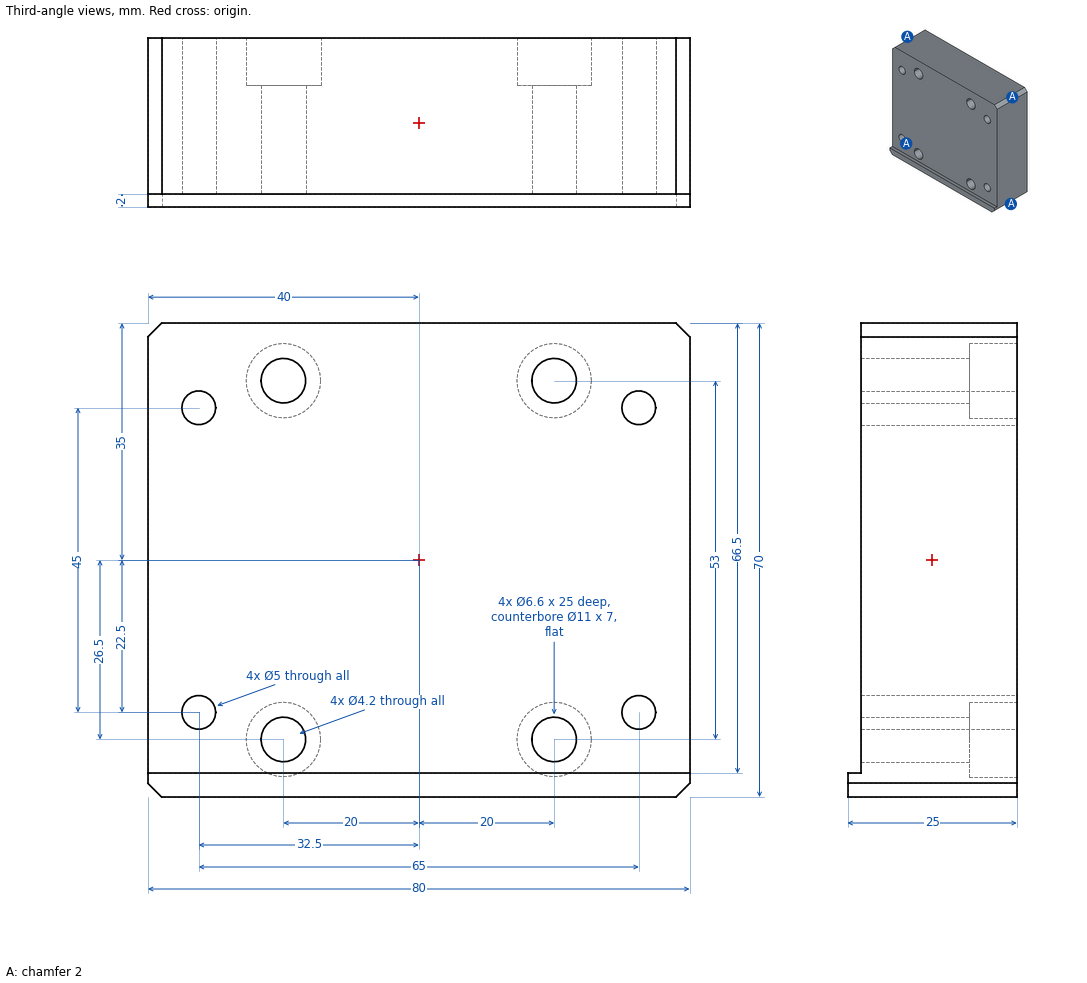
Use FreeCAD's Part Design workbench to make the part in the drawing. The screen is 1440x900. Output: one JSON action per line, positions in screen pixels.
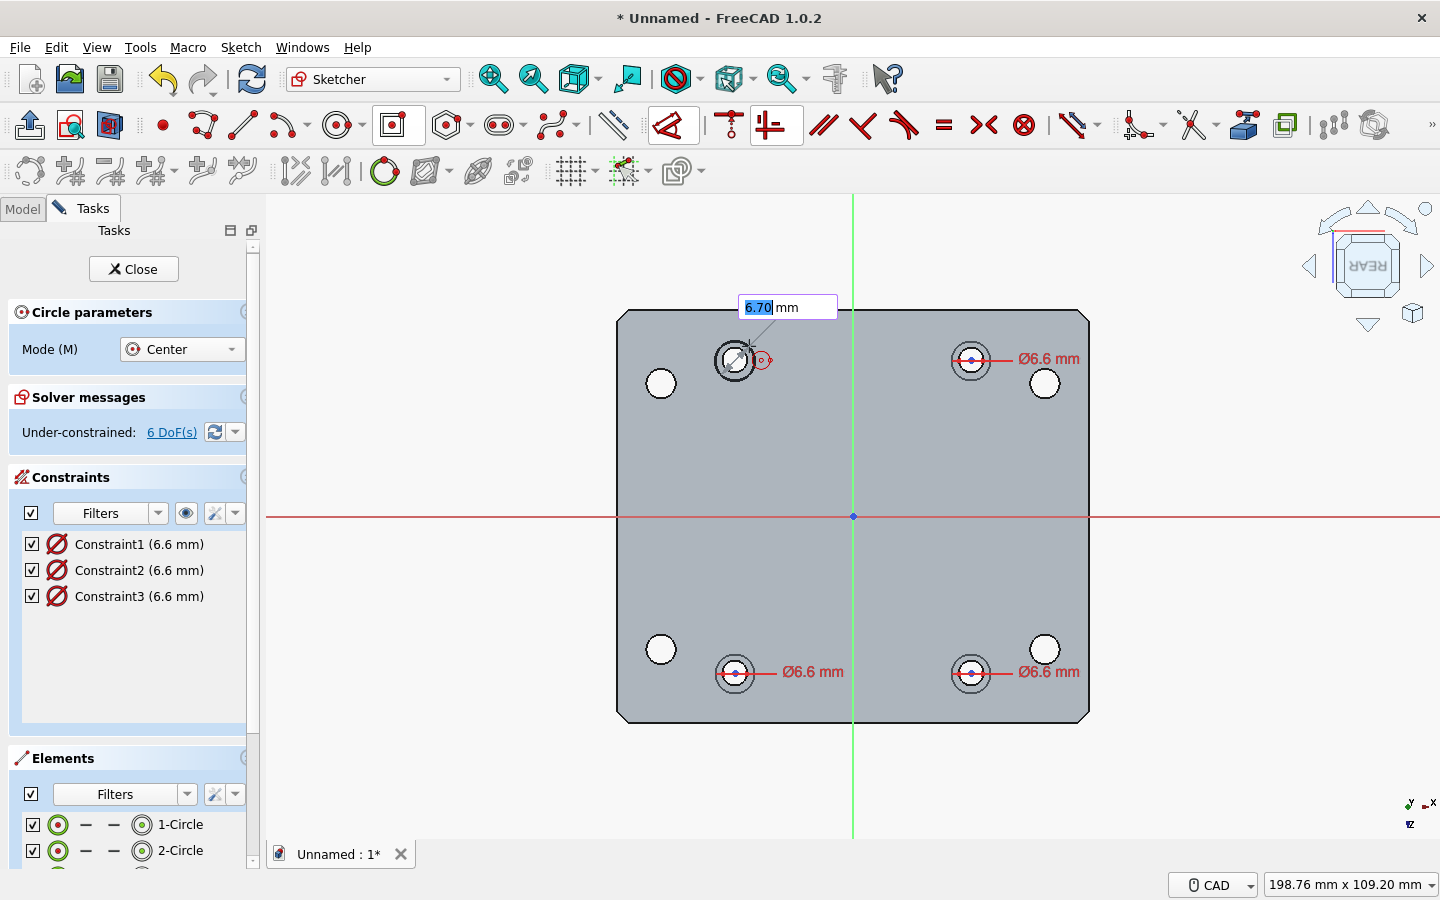
{"action": "type", "text": "6.6"}
{"action": "key", "text": "Return"}
{"action": "key", "text": "Escape"}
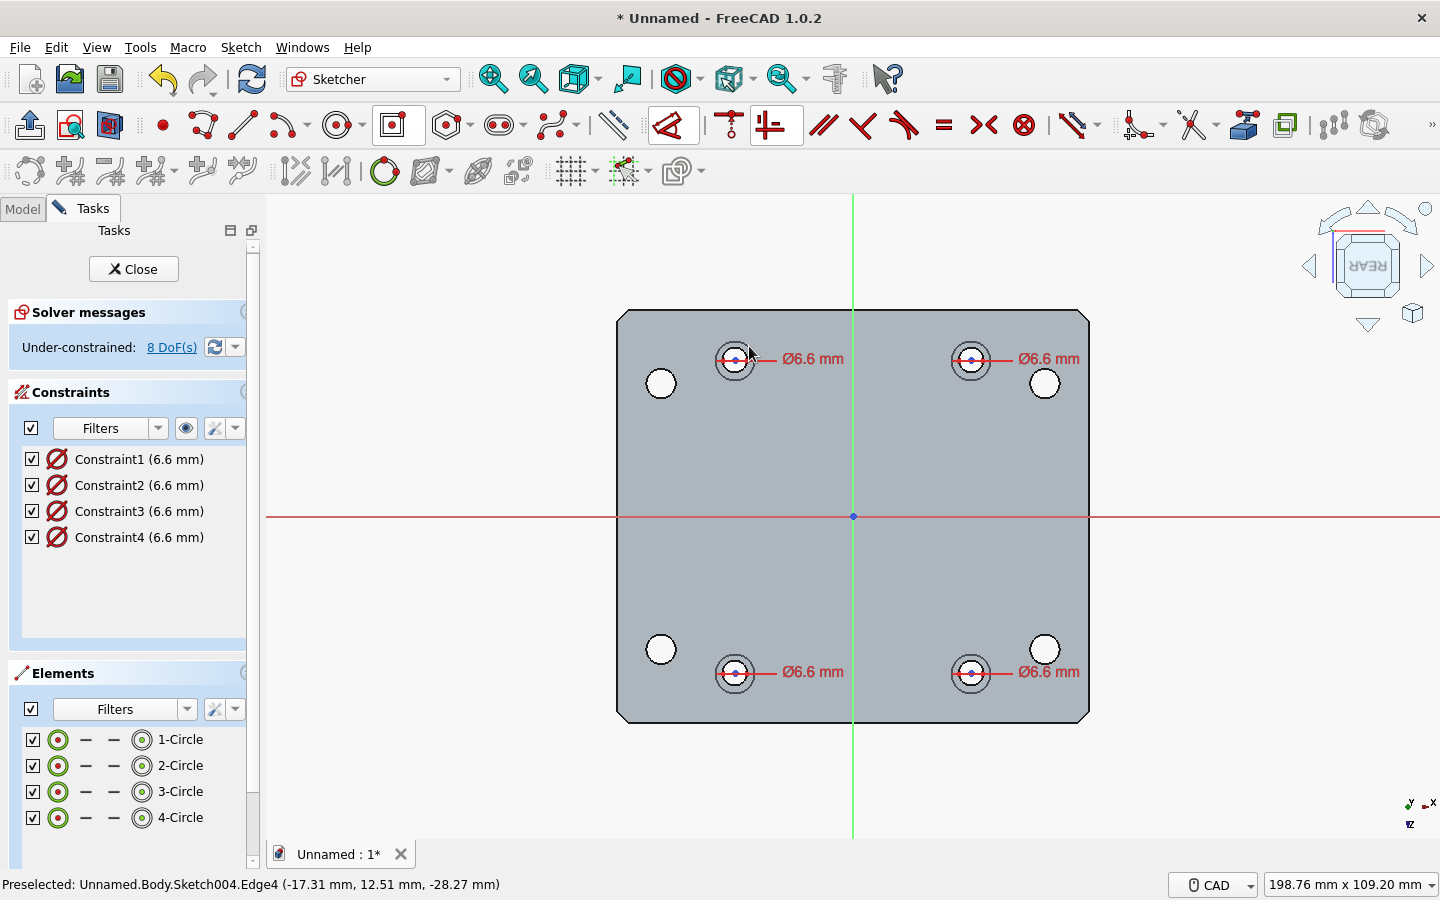
{"action": "left_click", "coordinate": [971, 361]}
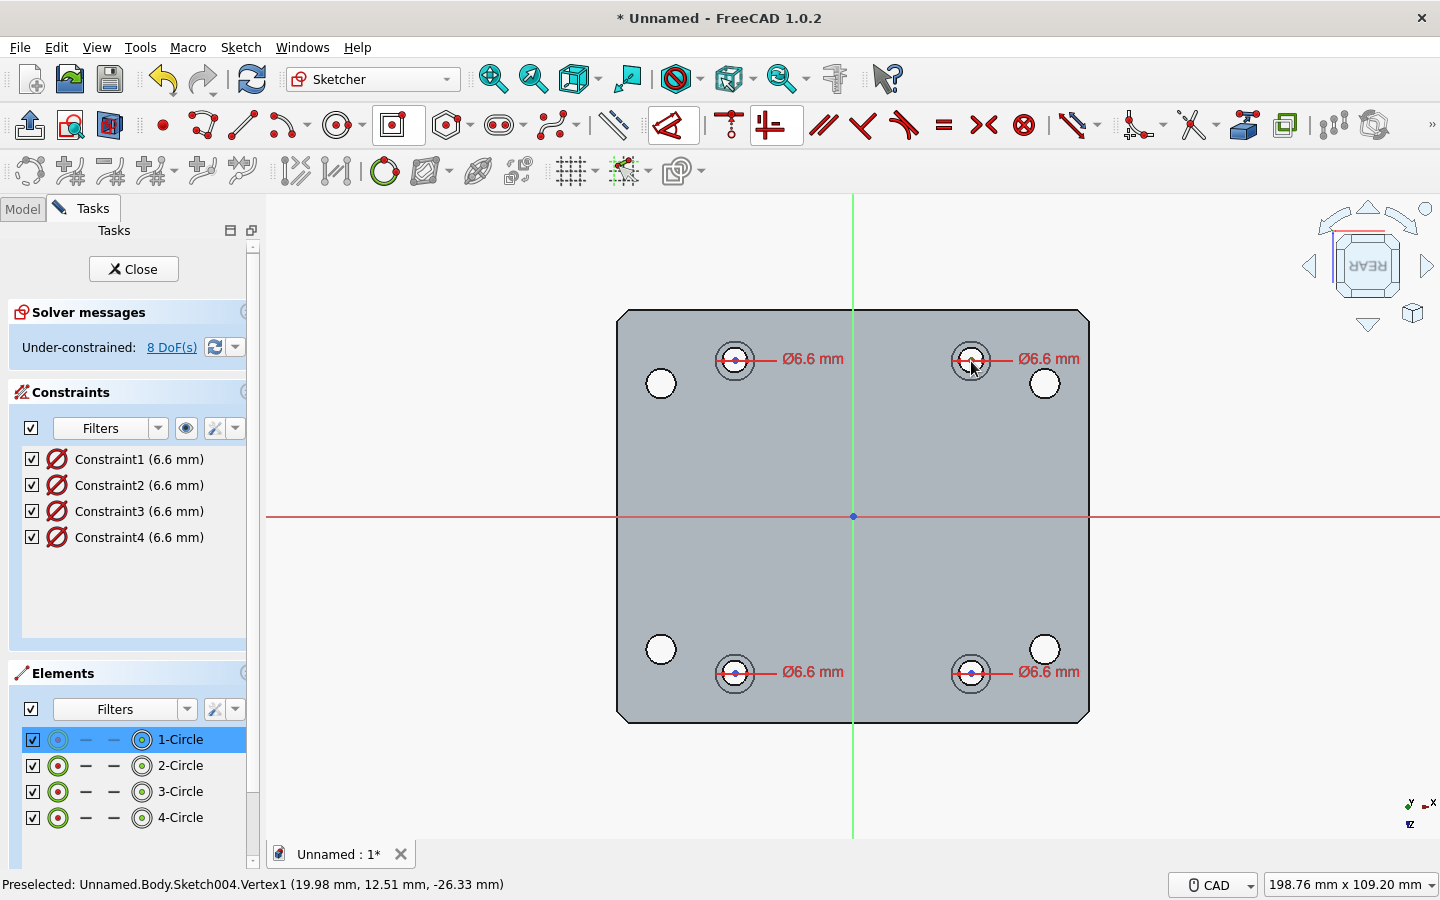
{"action": "left_click", "coordinate": [971, 674]}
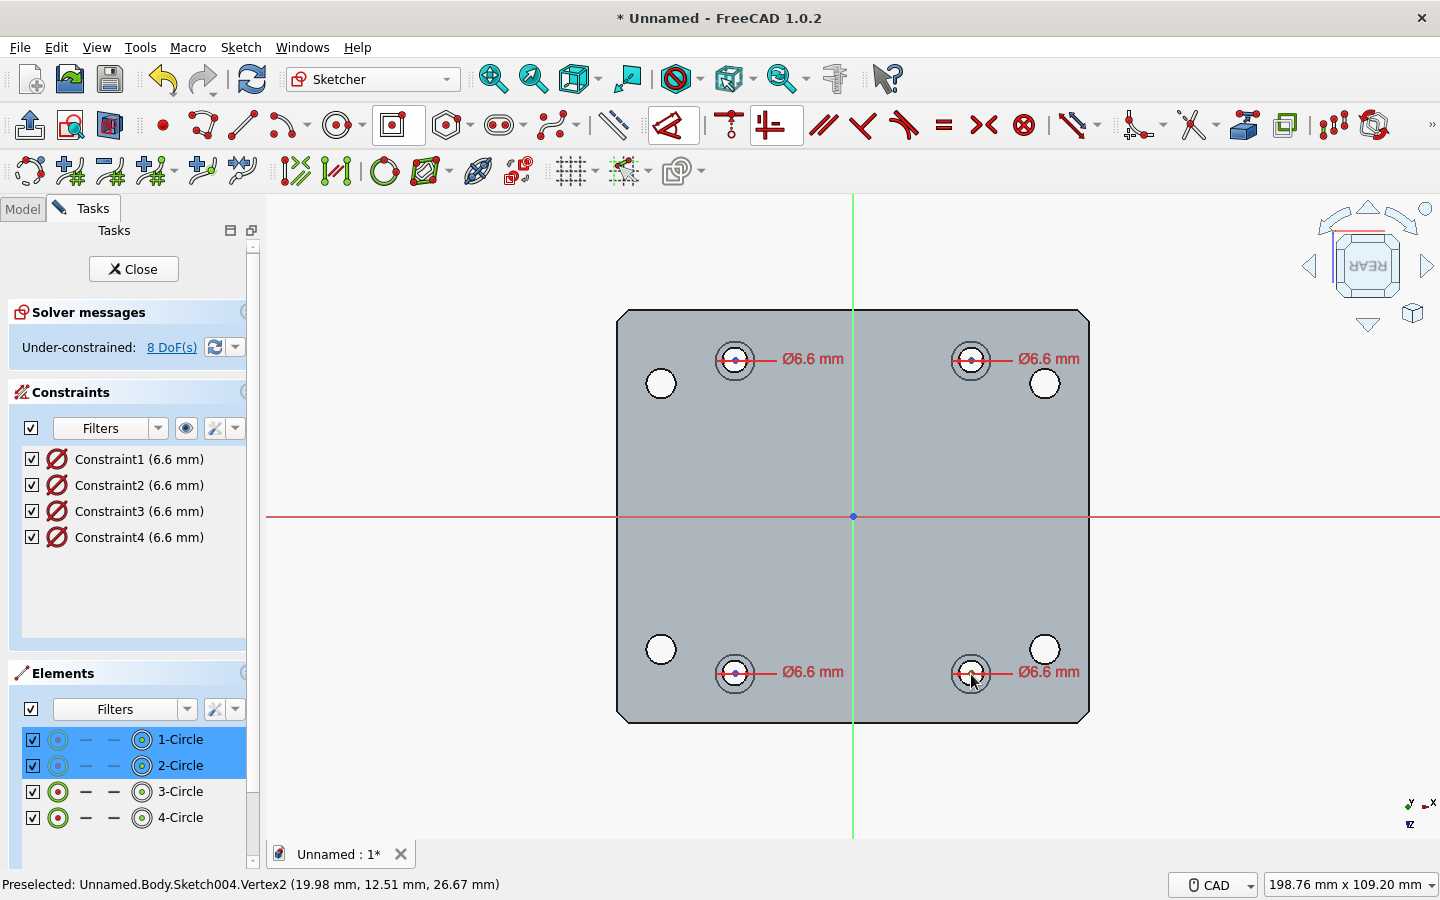
{"action": "key", "text": "v"}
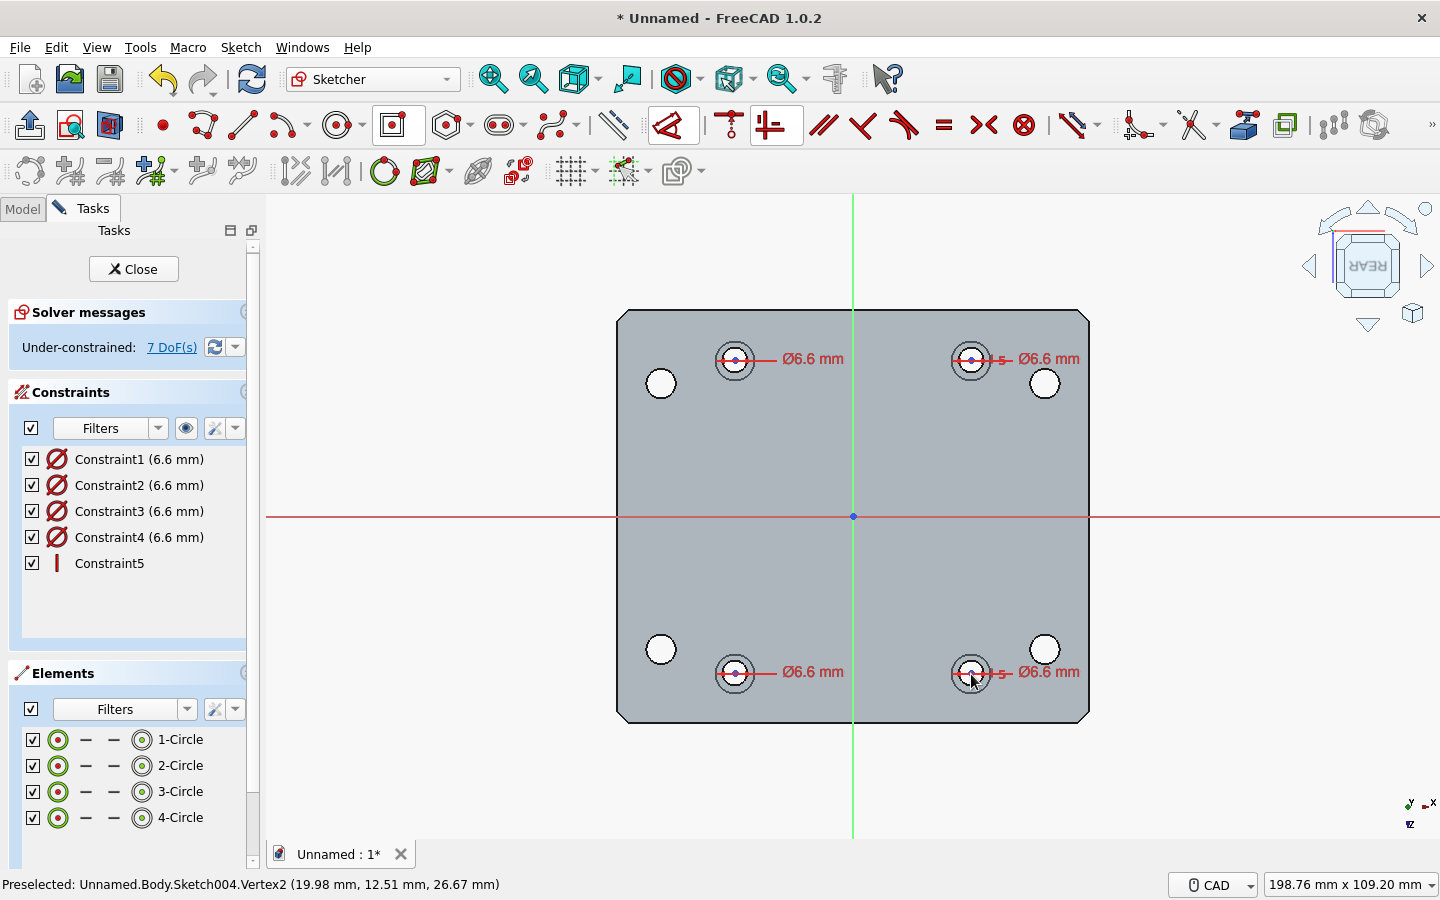
{"action": "left_click", "coordinate": [971, 674]}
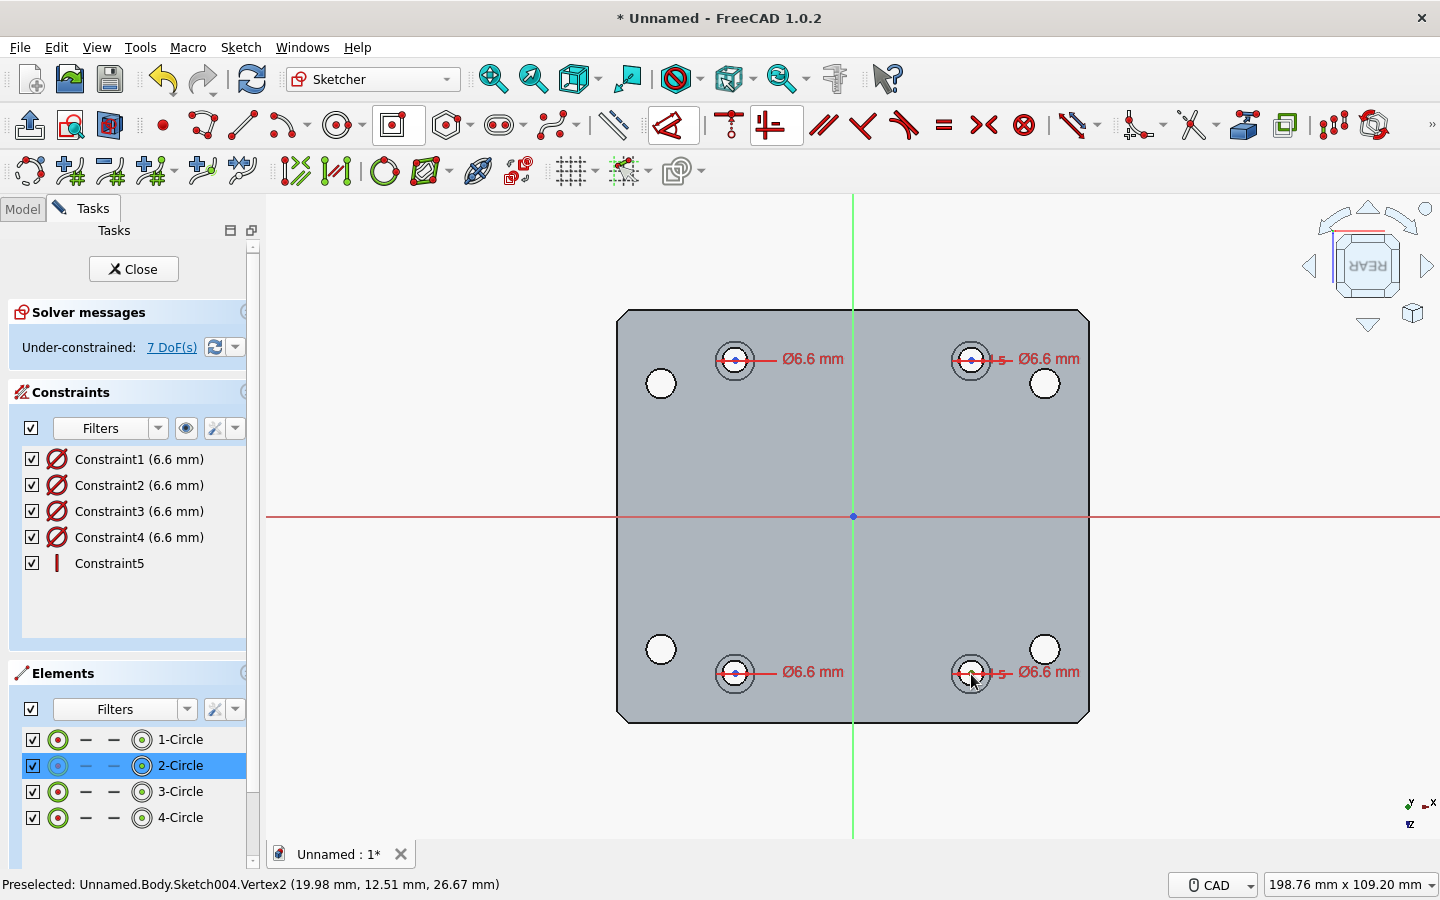
{"action": "left_click", "coordinate": [735, 674]}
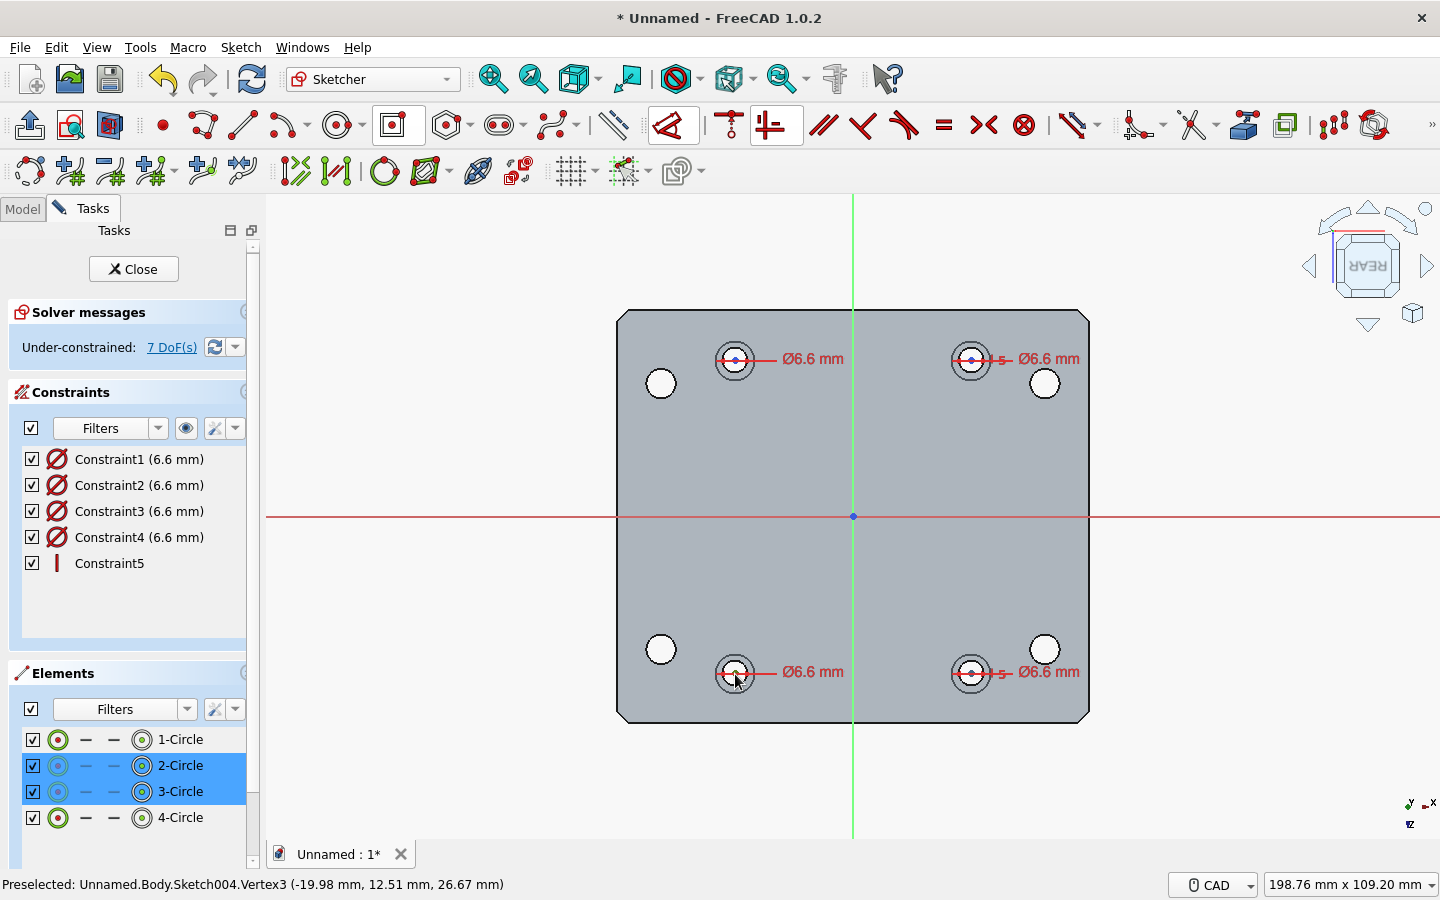
{"action": "left_click", "coordinate": [798, 126]}